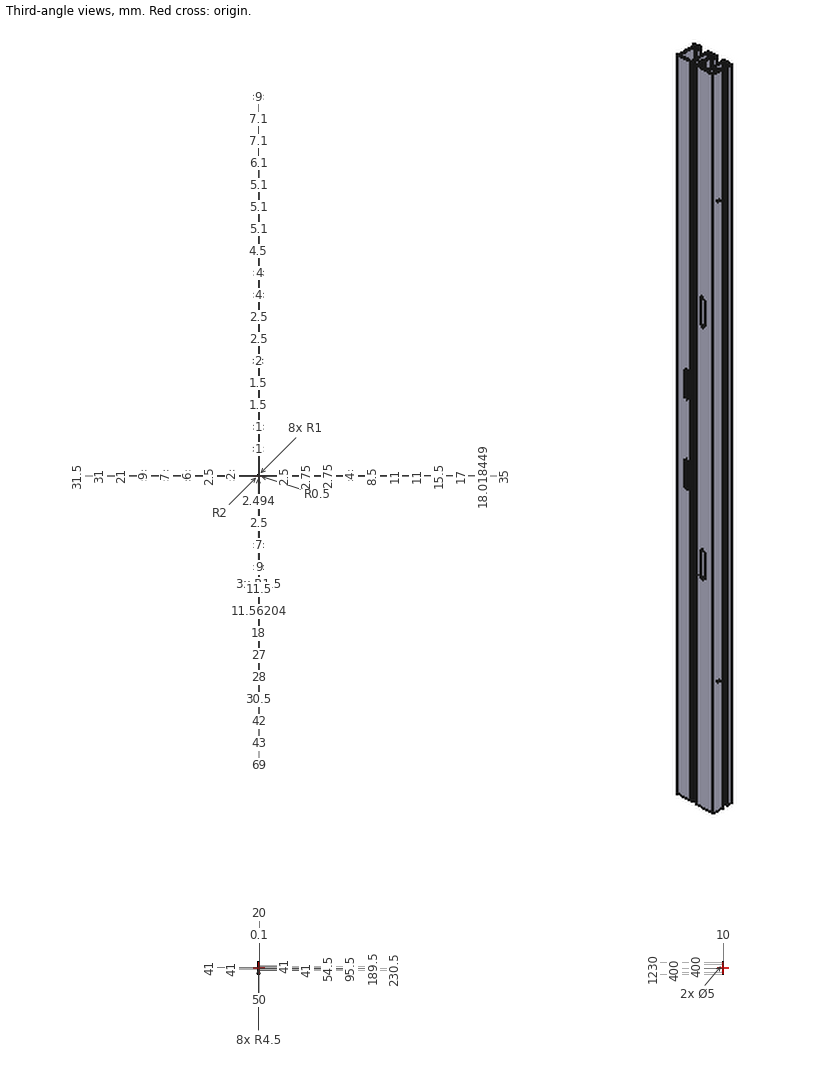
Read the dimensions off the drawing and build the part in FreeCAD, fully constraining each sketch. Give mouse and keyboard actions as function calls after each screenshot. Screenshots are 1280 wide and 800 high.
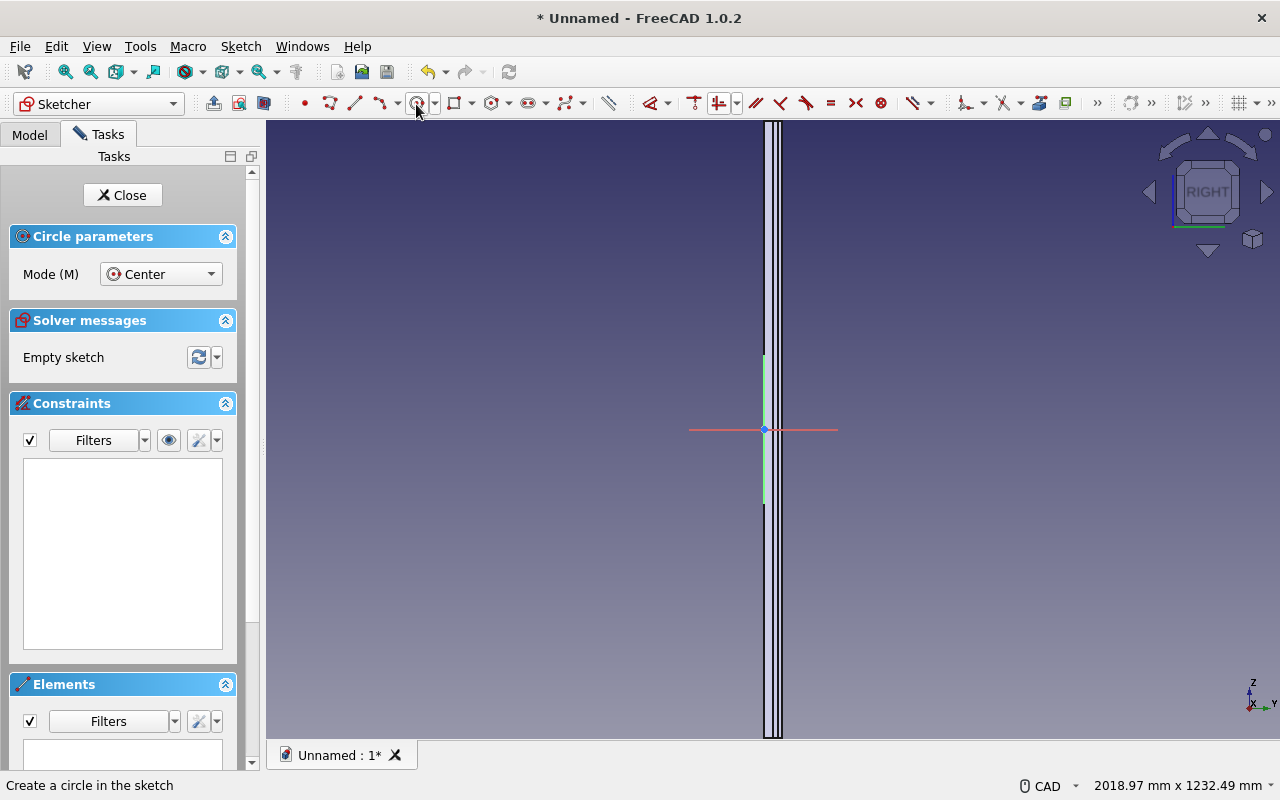
scroll(769, 229, up, 15)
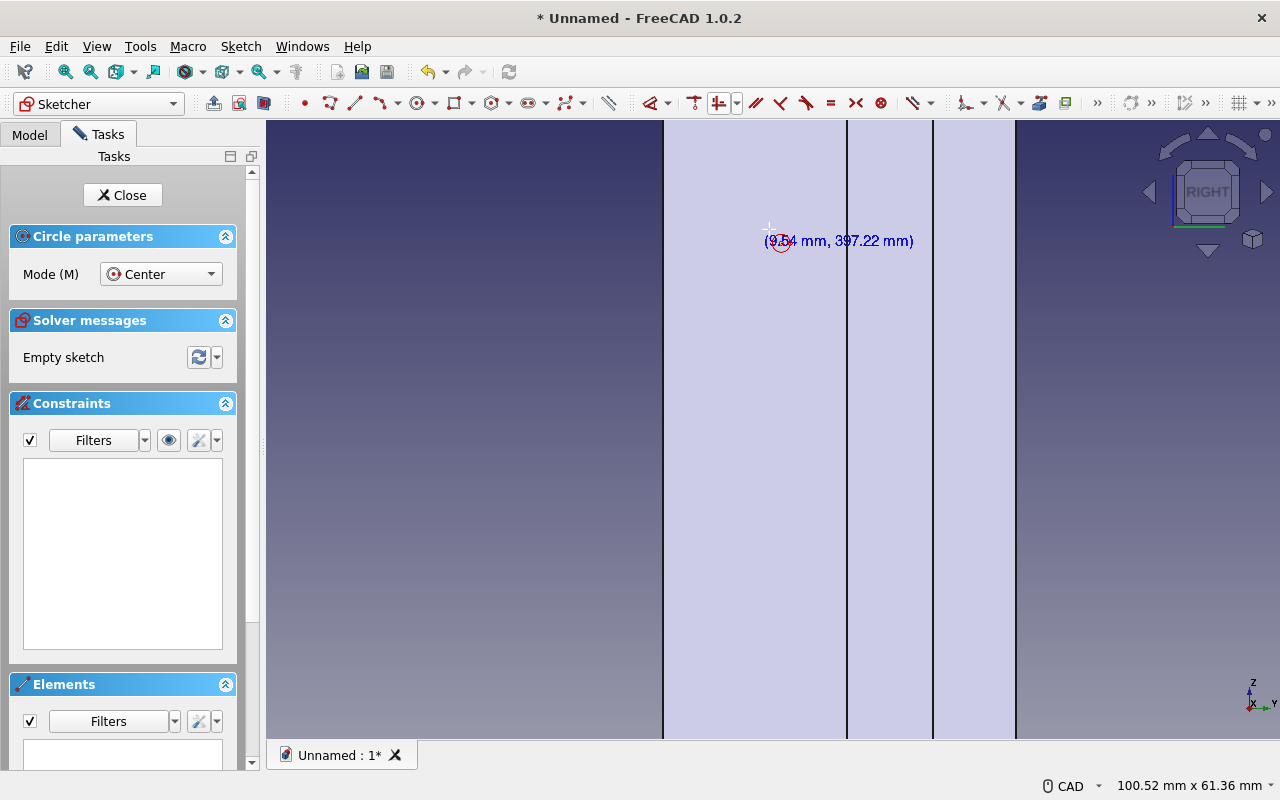
scroll(703, 229, down, 15)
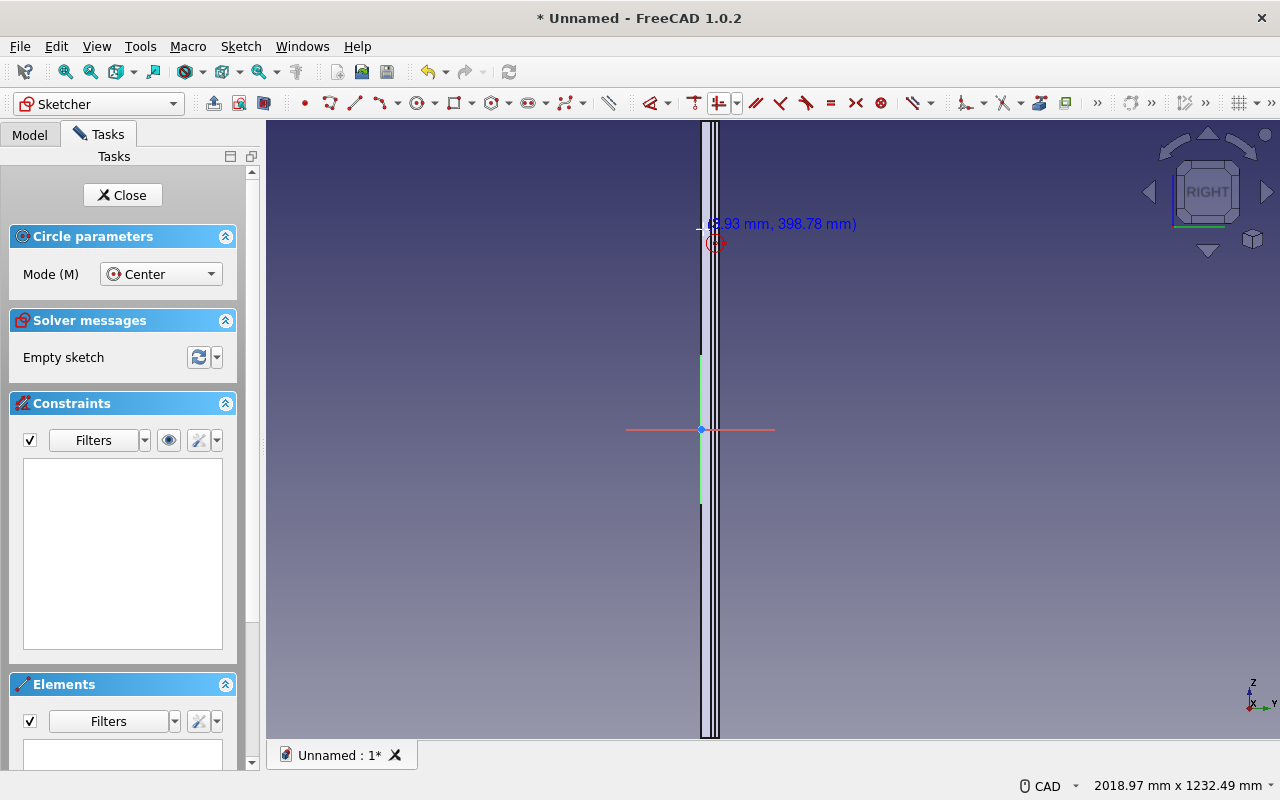
scroll(706, 229, up, 6)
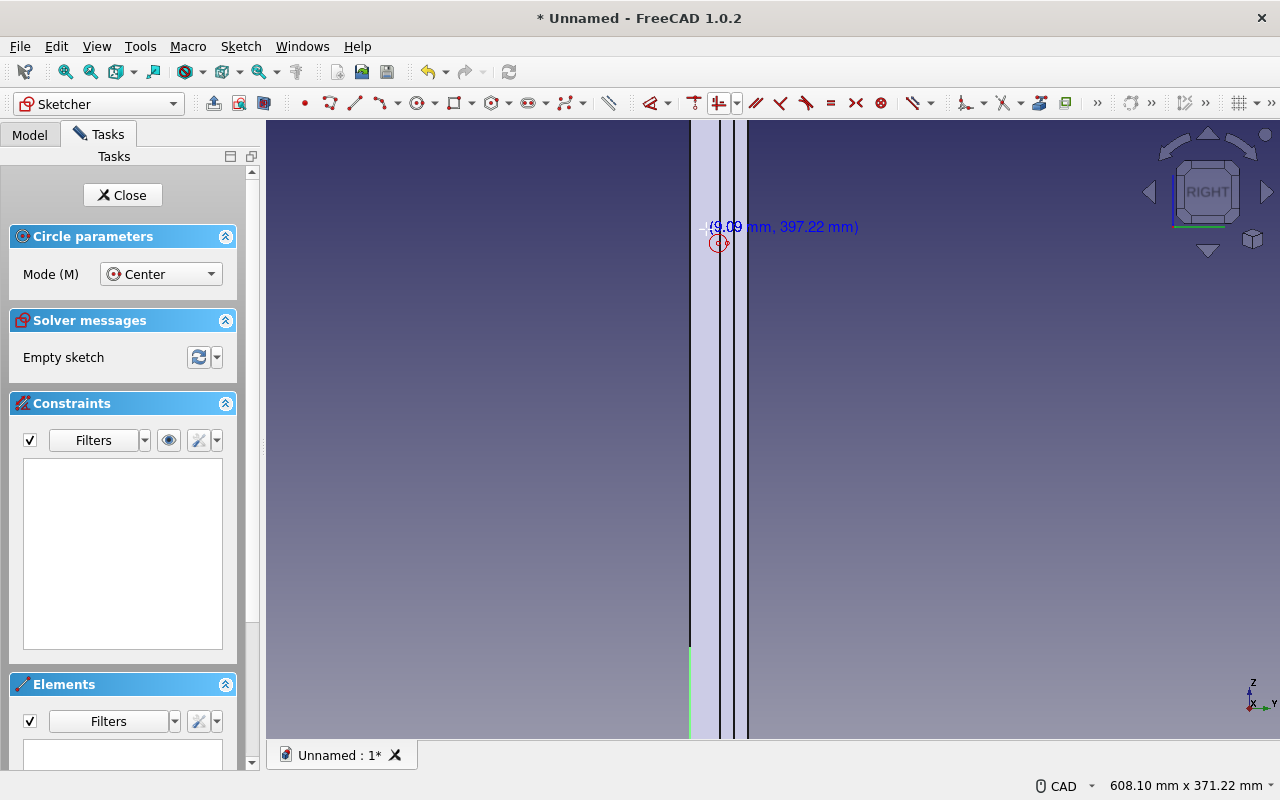
click(707, 227)
move(709, 224)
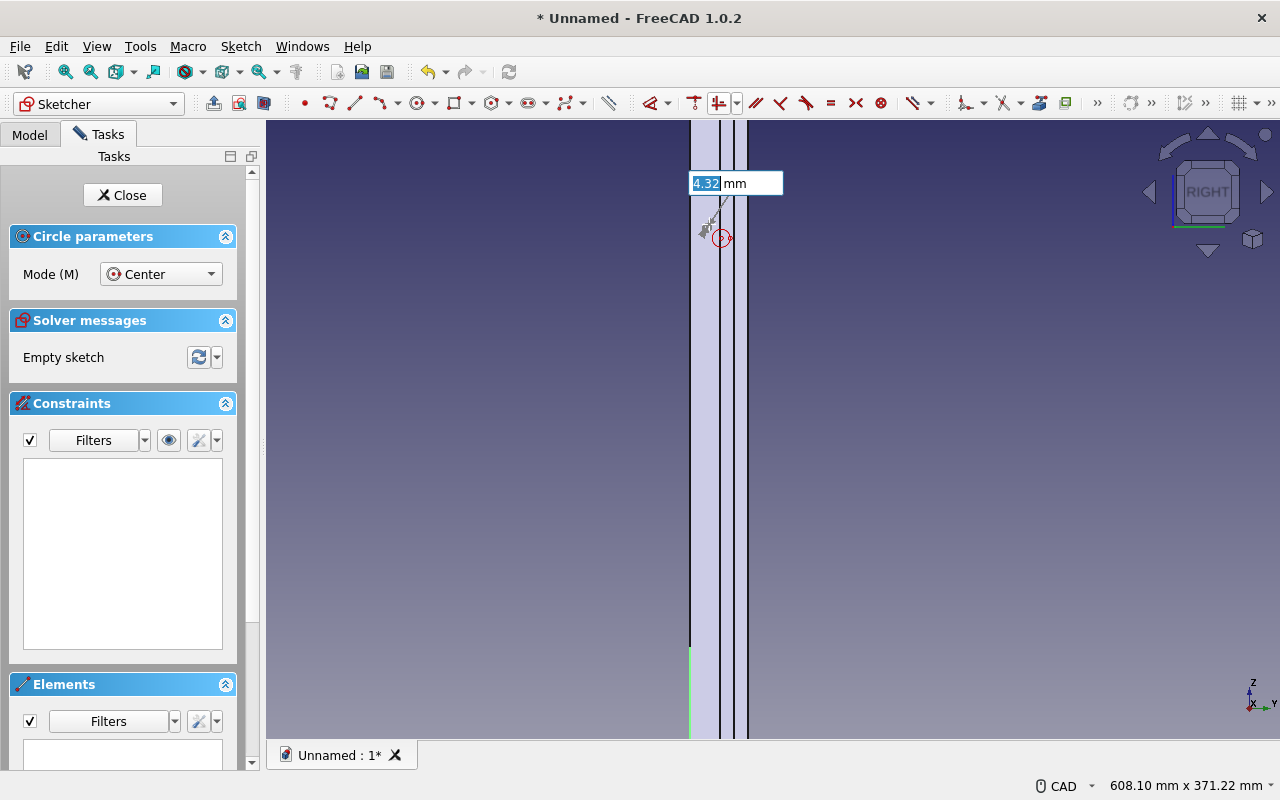
text(5)
key(Return)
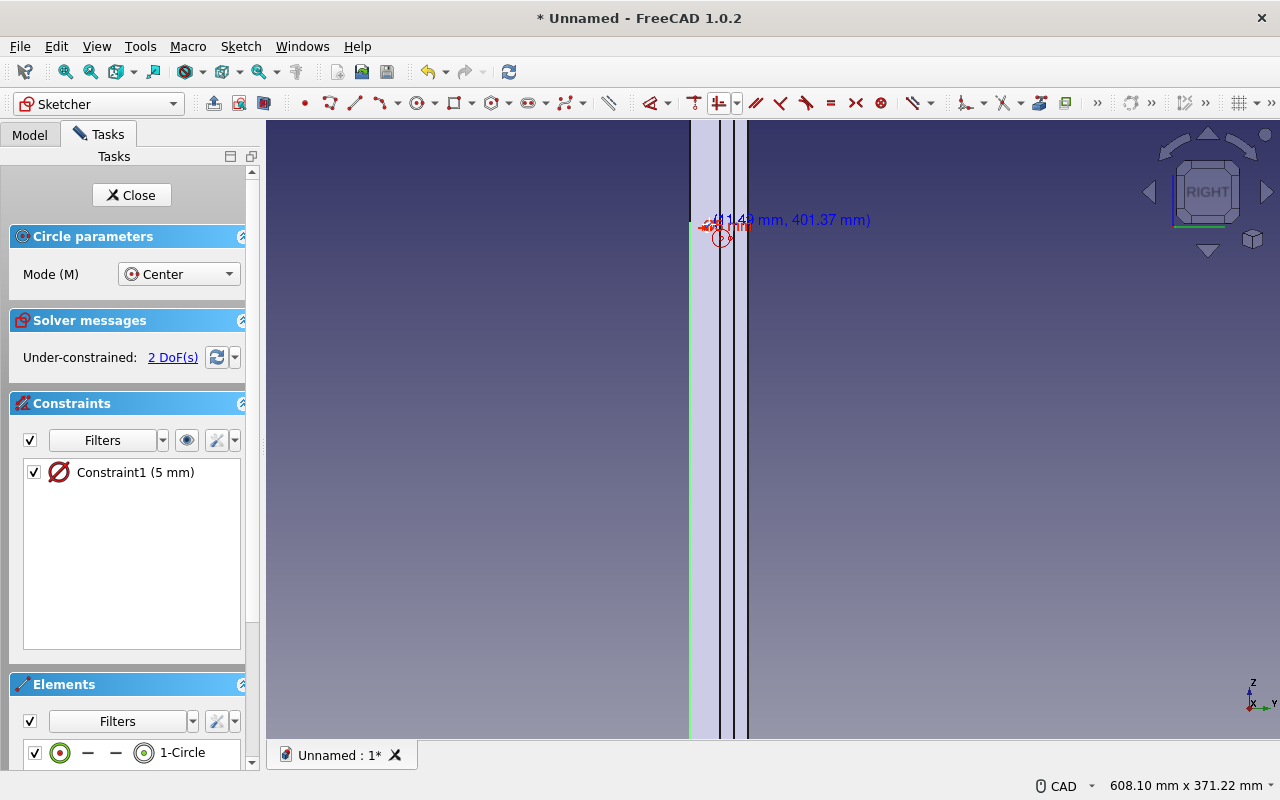
scroll(706, 229, down, 6)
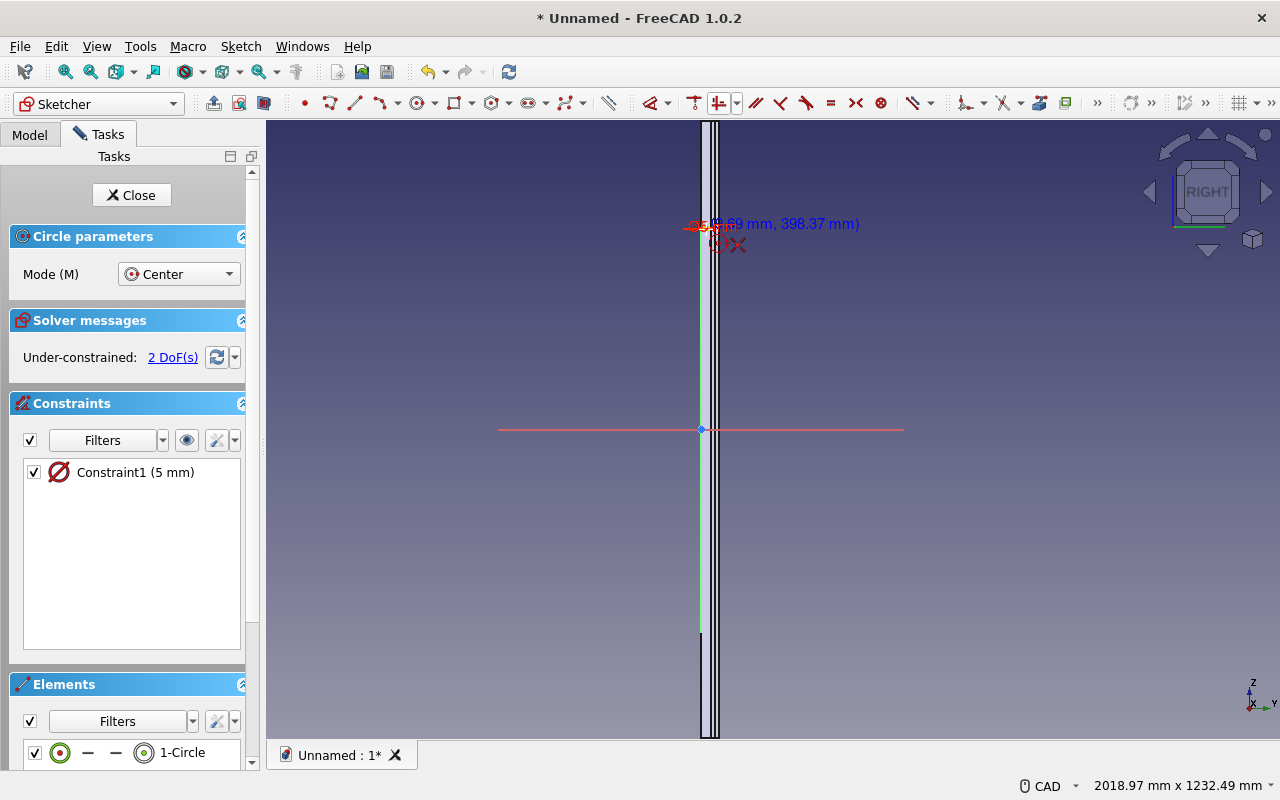
scroll(706, 630, up, 15)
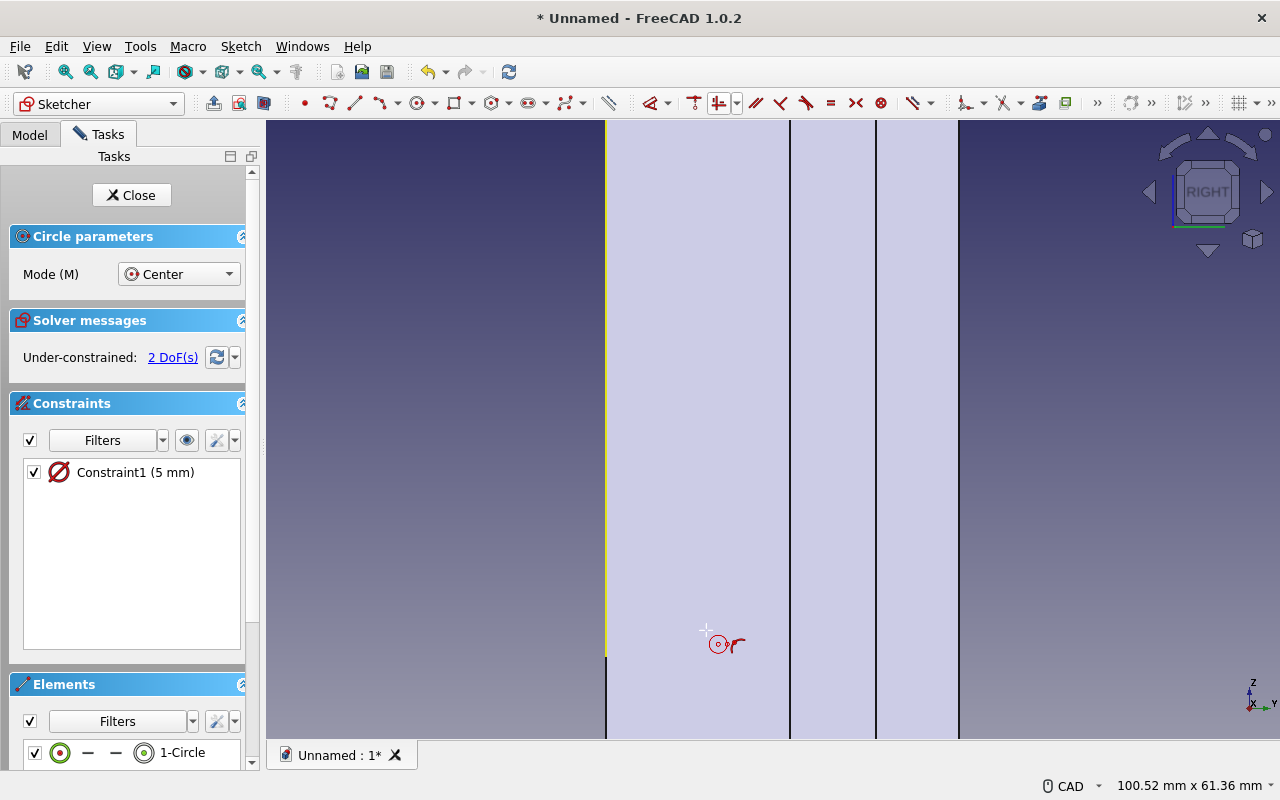
scroll(706, 631, down, 15)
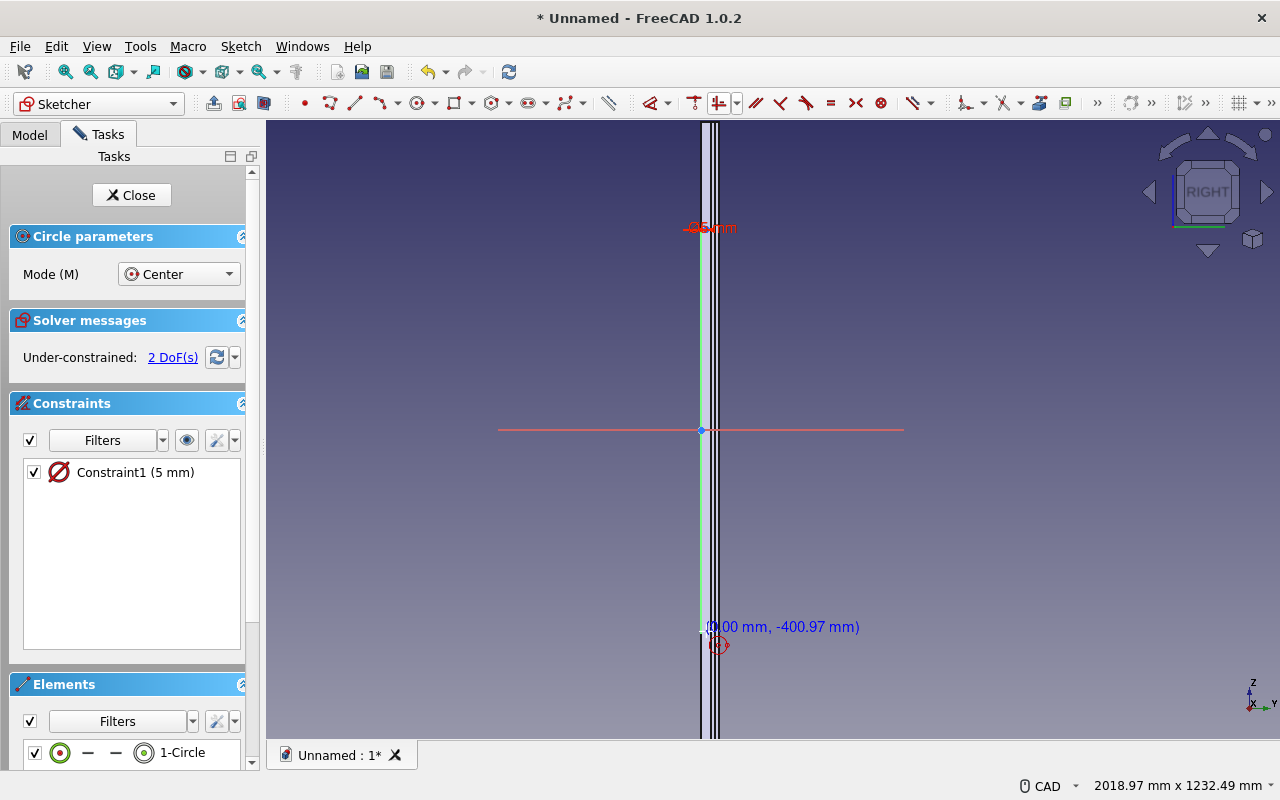
scroll(706, 631, up, 6)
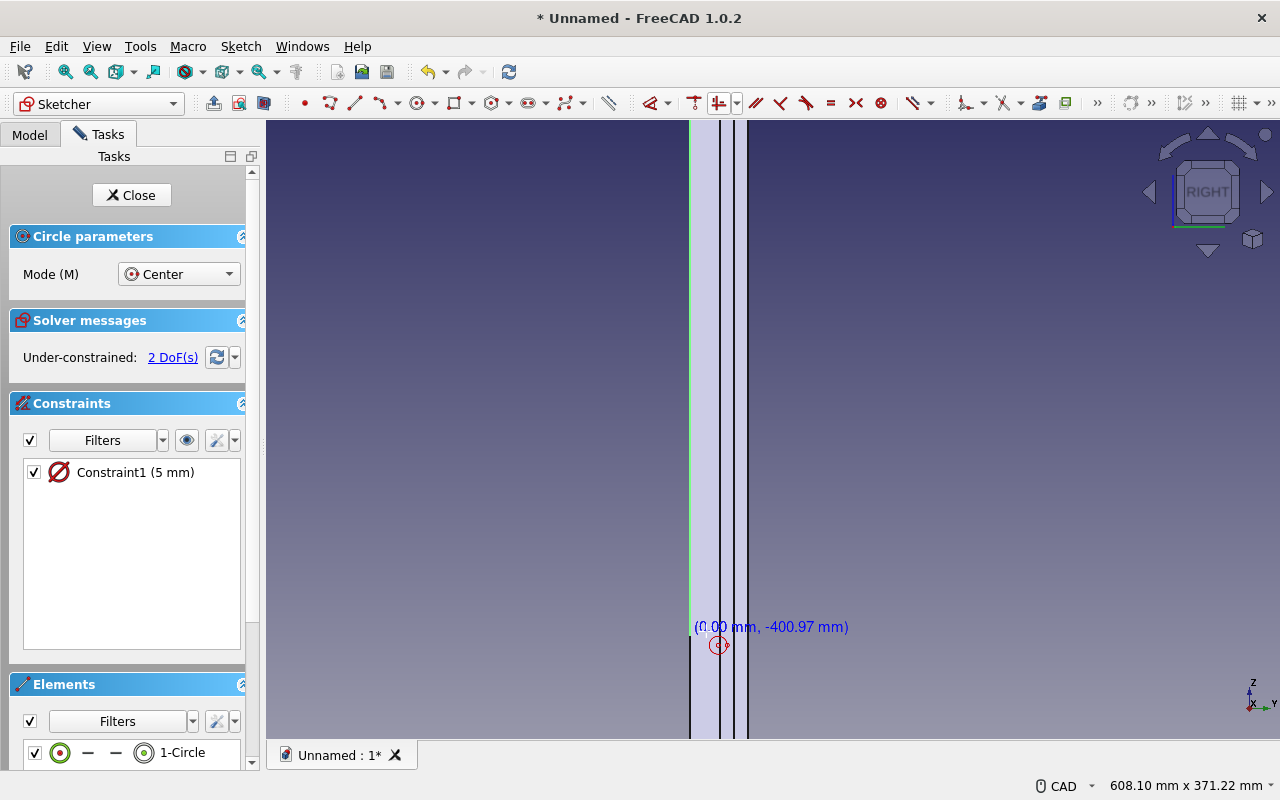
click(707, 630)
move(709, 627)